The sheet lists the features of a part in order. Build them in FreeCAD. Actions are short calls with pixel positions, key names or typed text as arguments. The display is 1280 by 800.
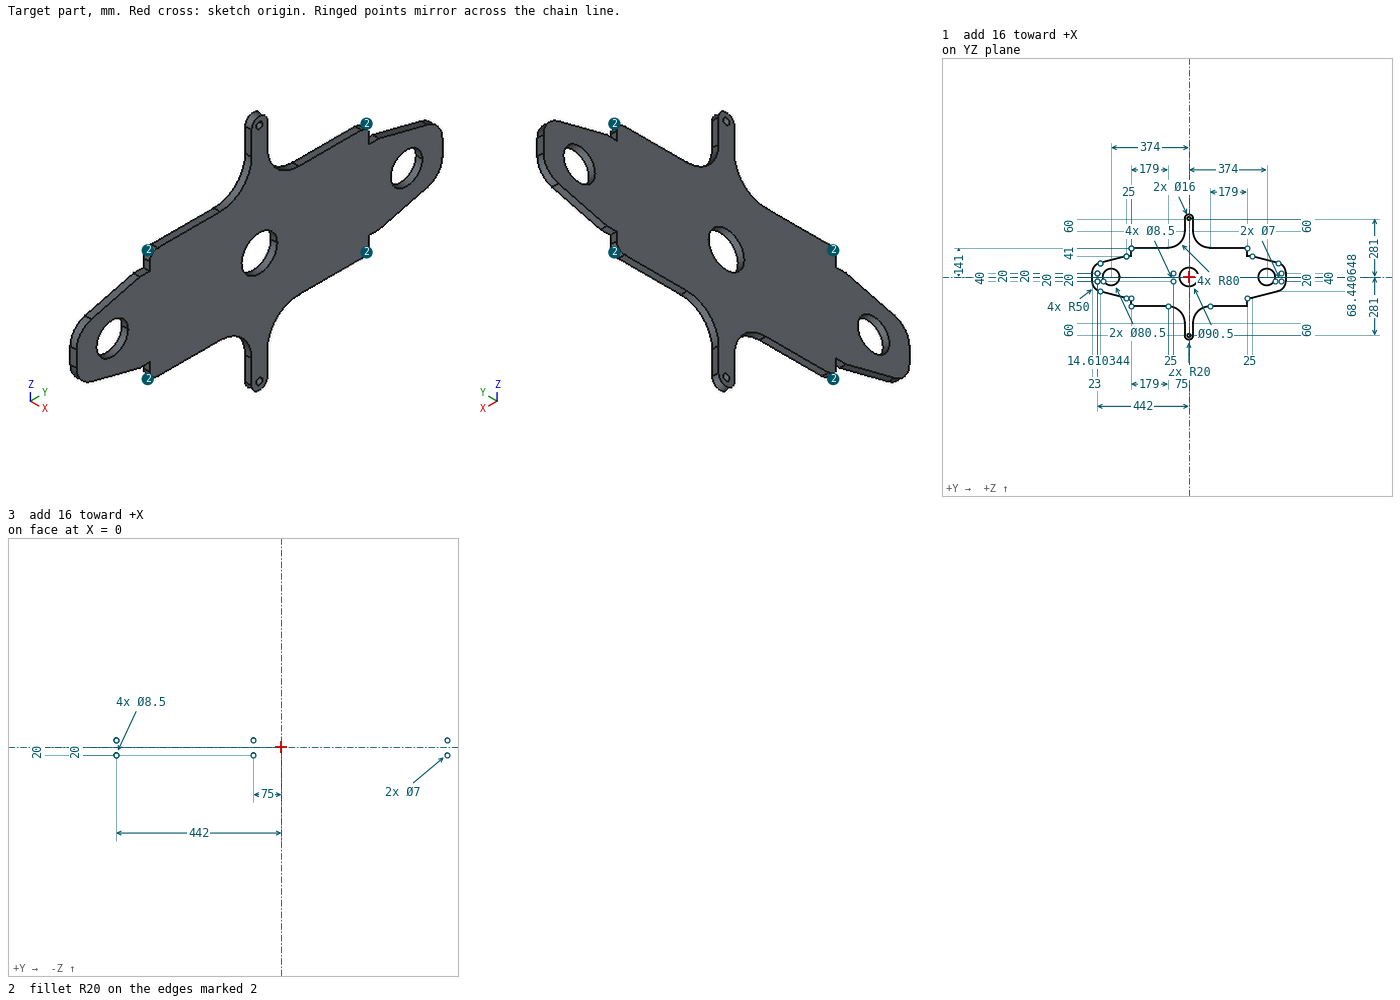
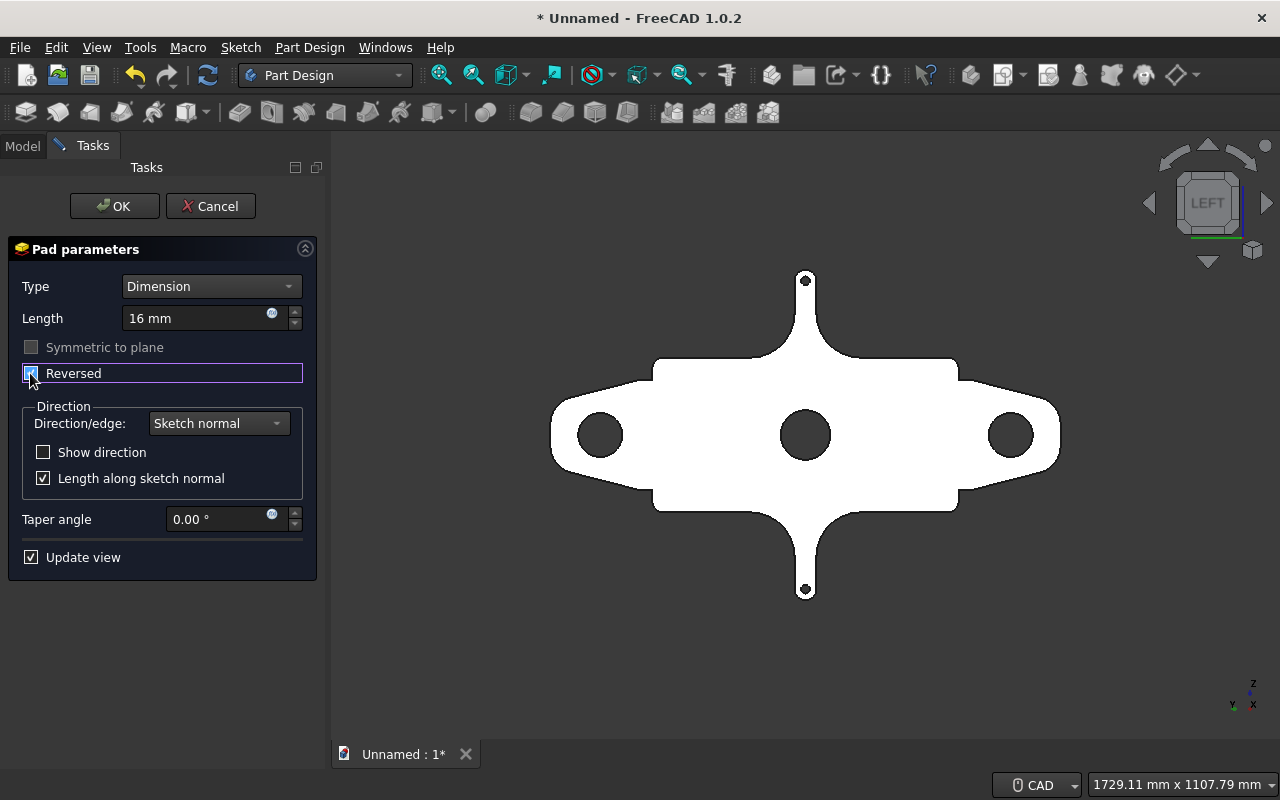
click(115, 206)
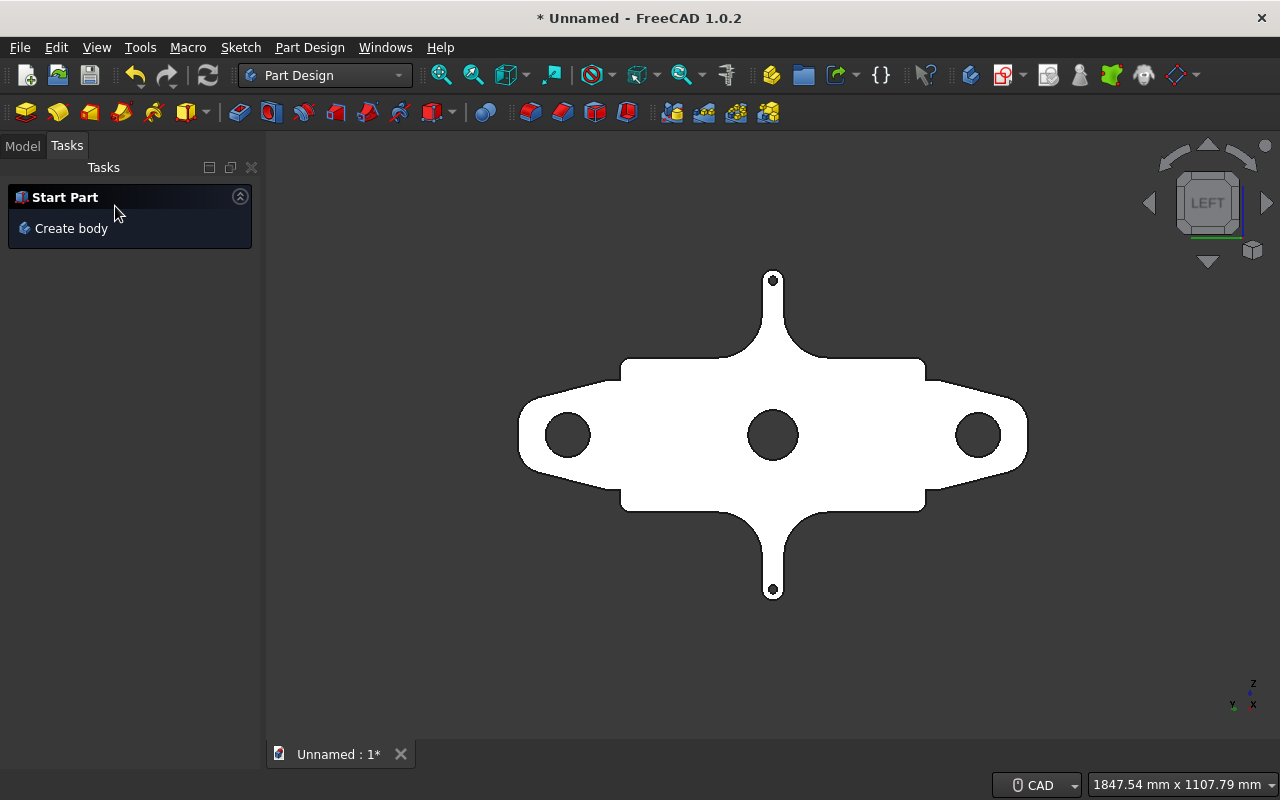
key(0)